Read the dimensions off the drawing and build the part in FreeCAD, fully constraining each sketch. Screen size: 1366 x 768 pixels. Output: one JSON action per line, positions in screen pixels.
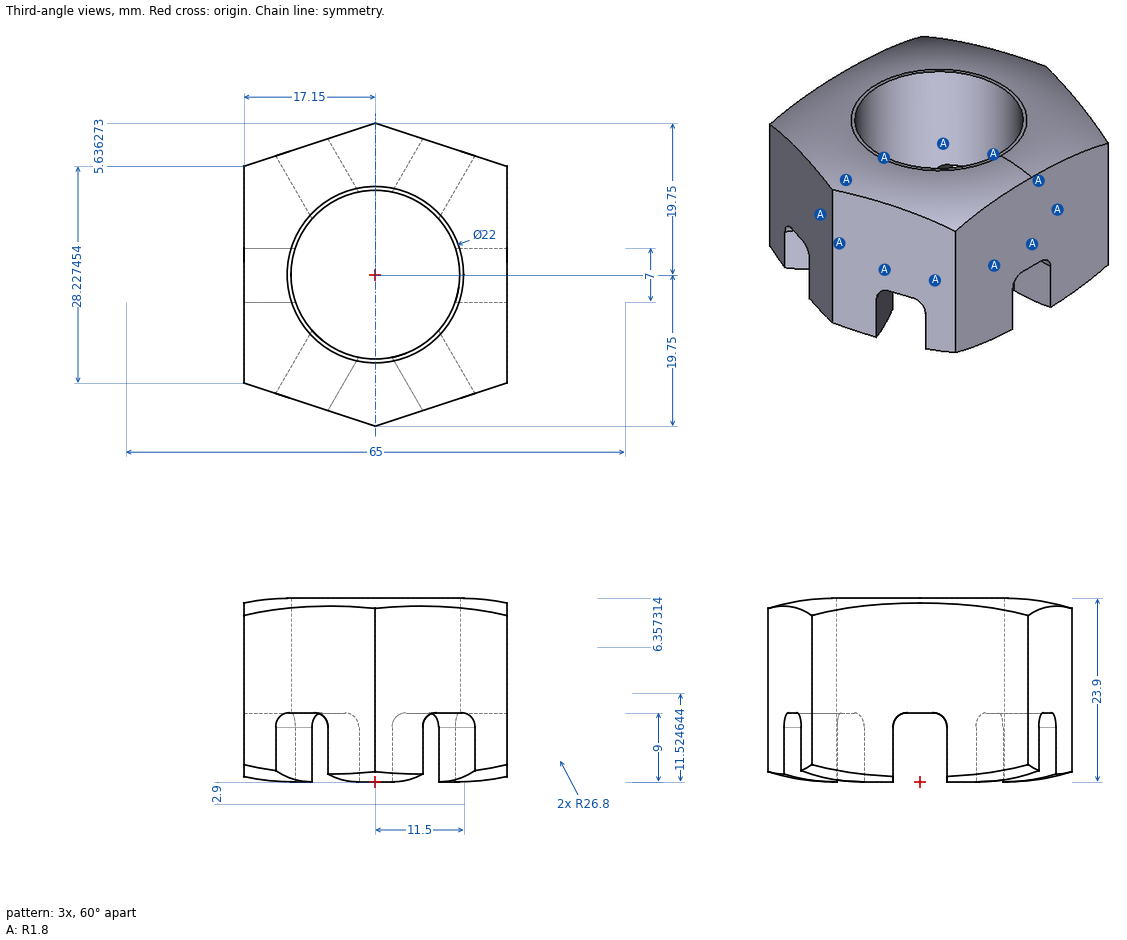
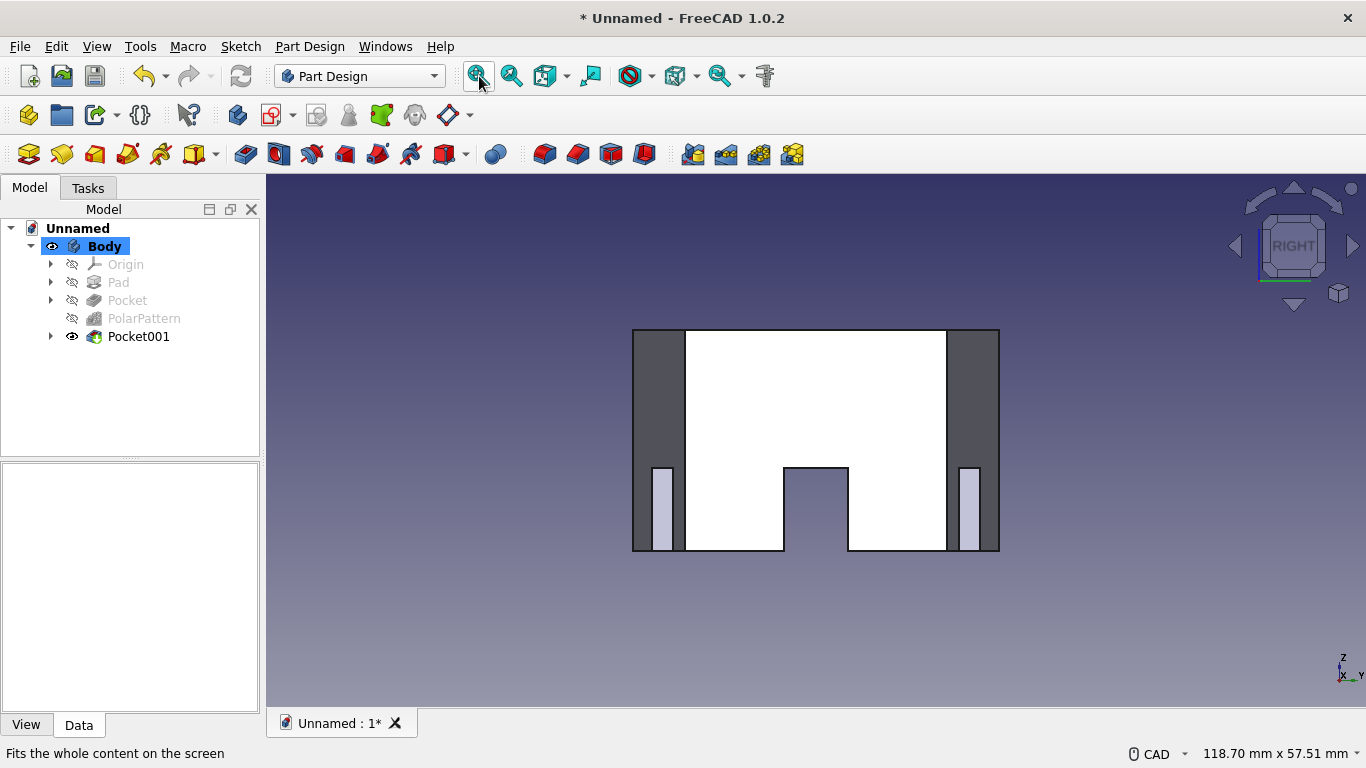
{"action": "key", "text": "5"}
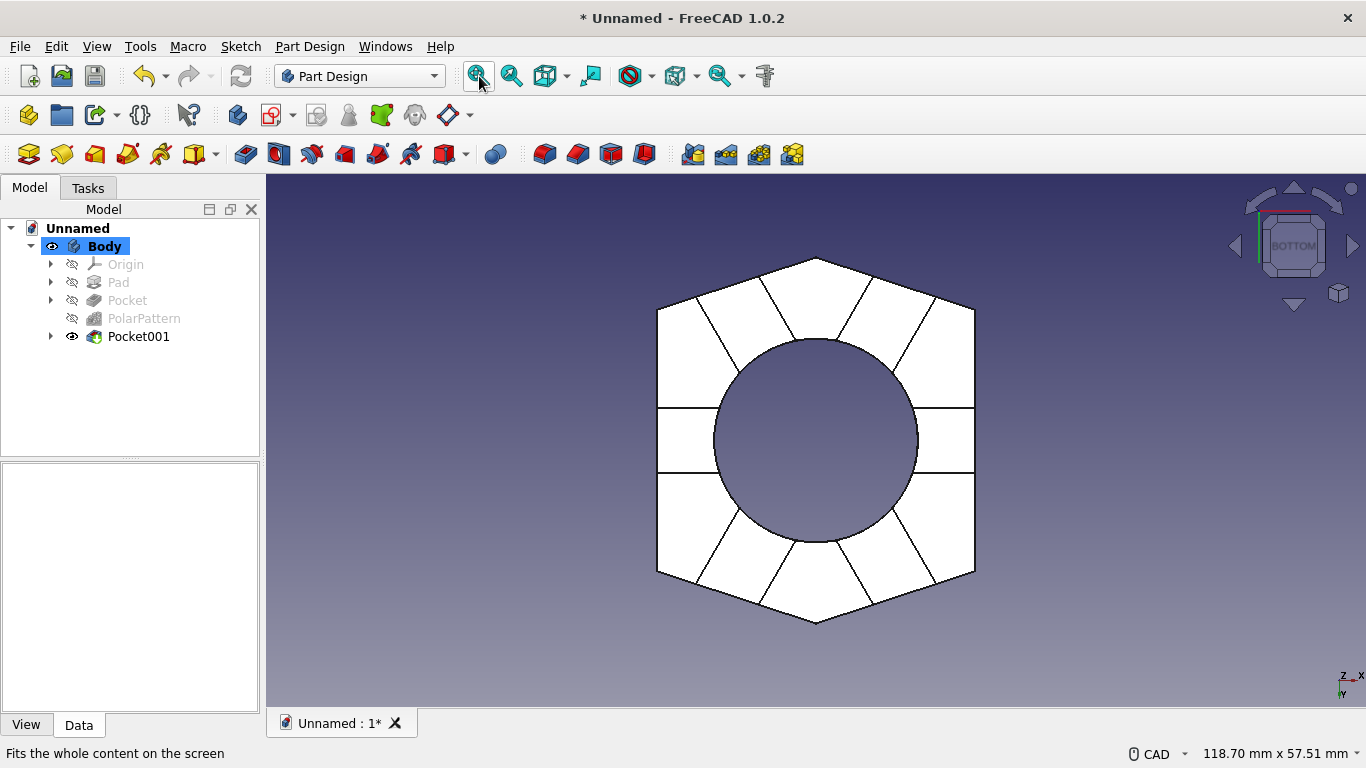
{"action": "key", "text": "4"}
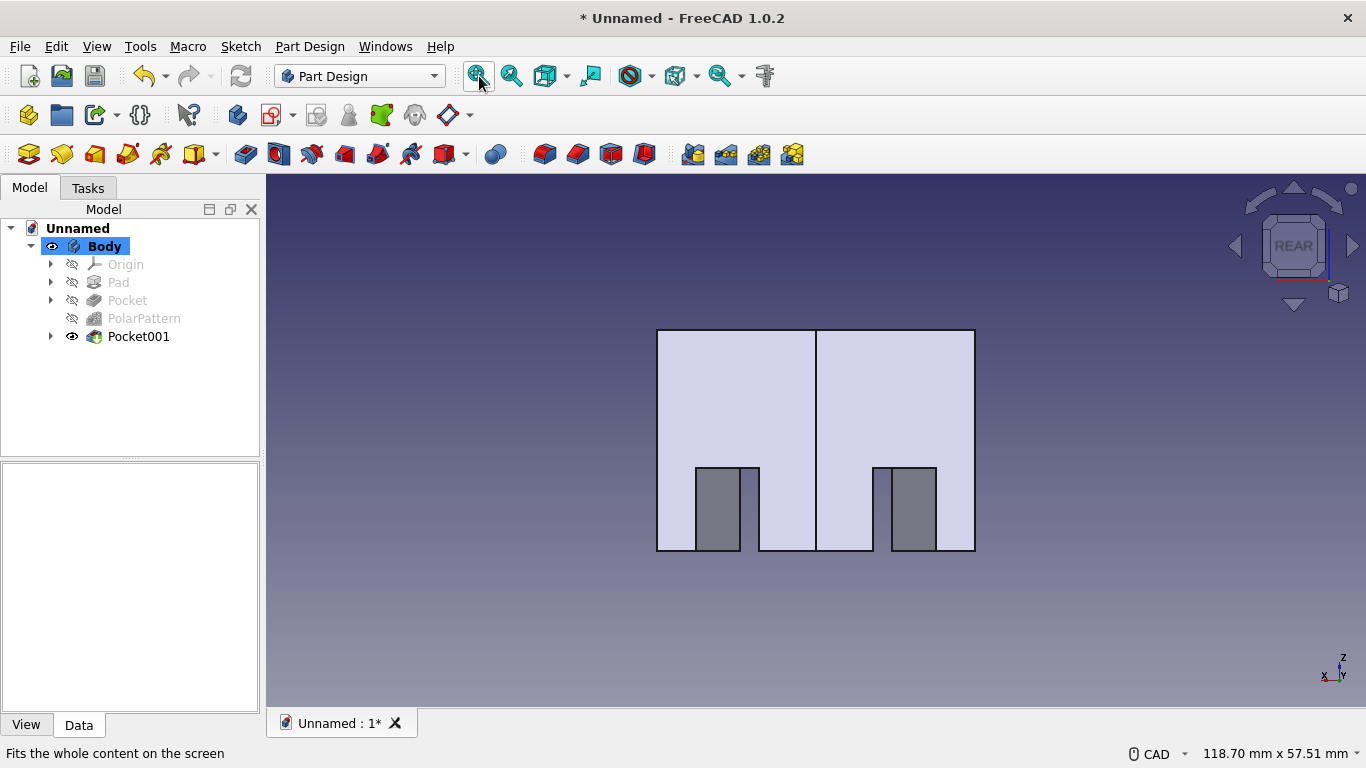
{"action": "left_click", "coordinate": [479, 76]}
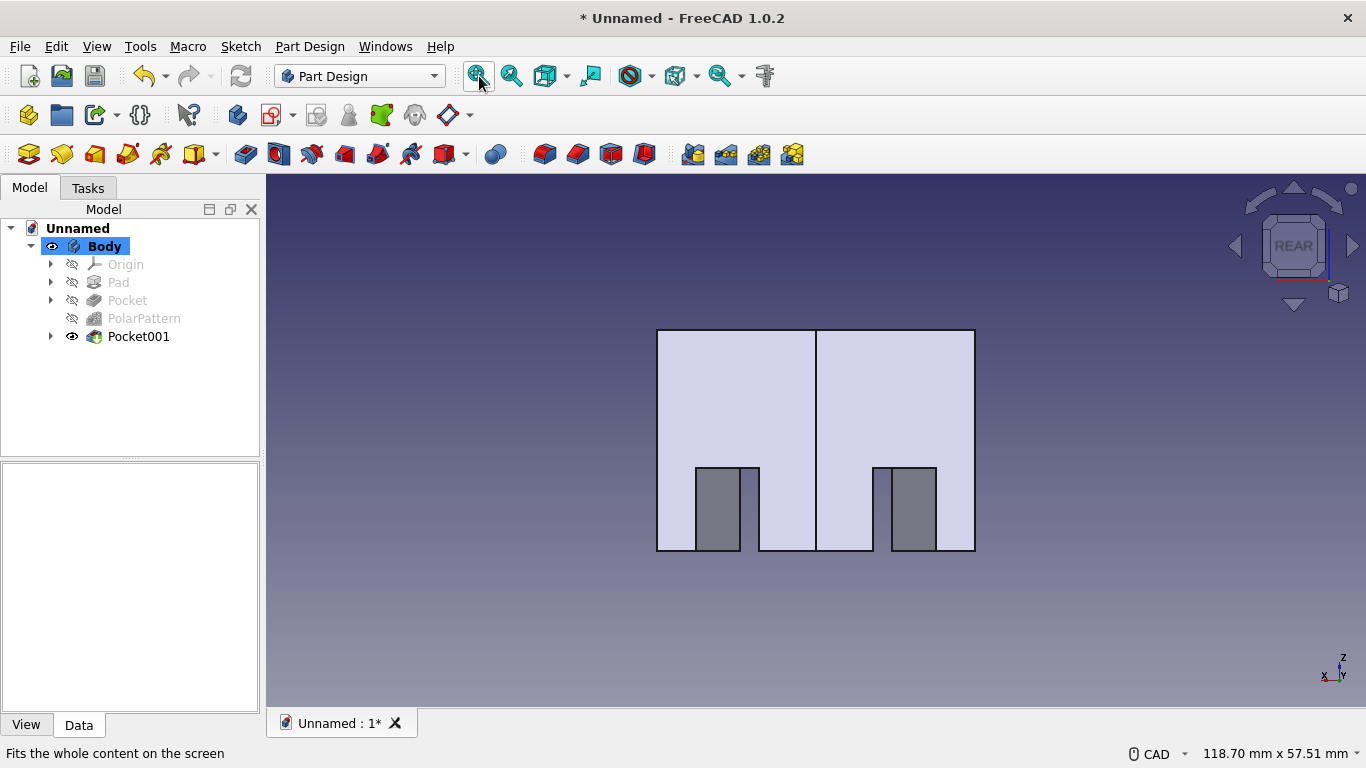
{"action": "key", "text": "6"}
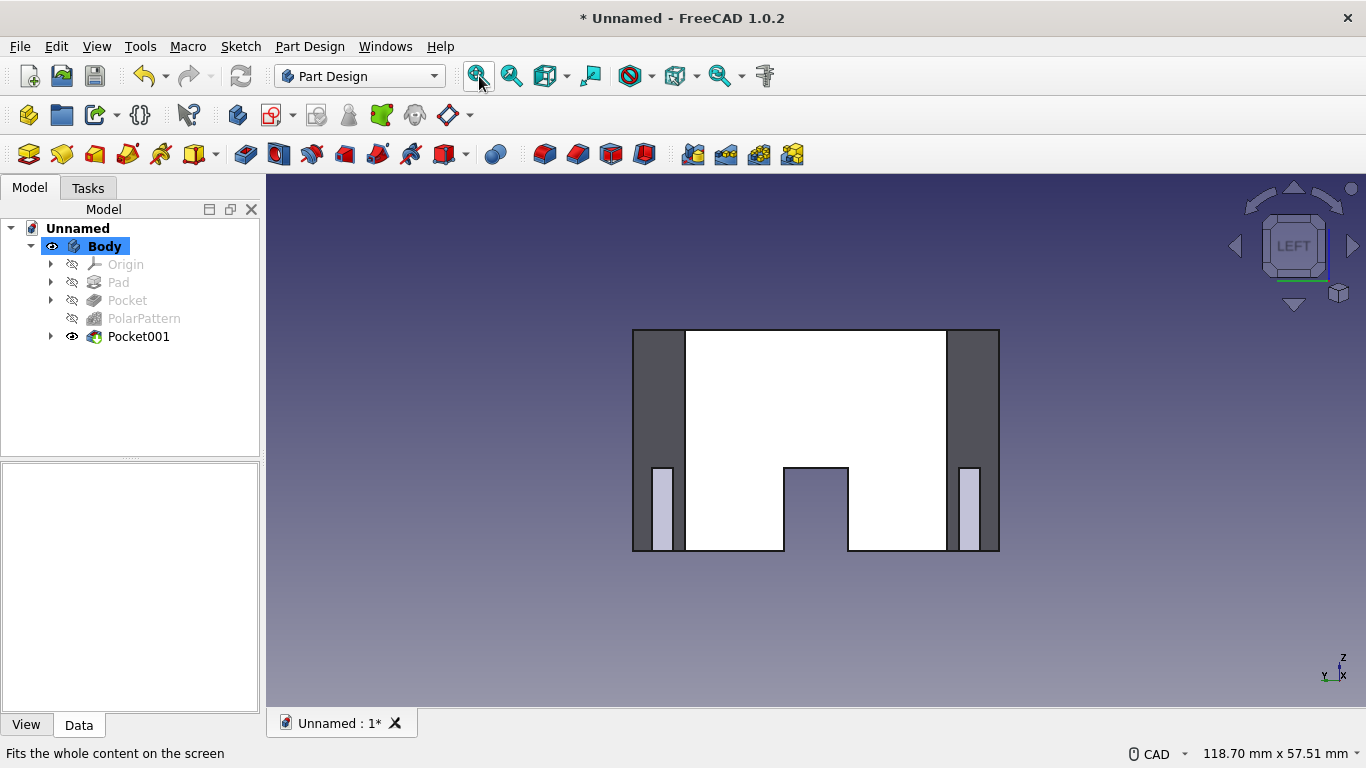
{"action": "left_click", "coordinate": [479, 76]}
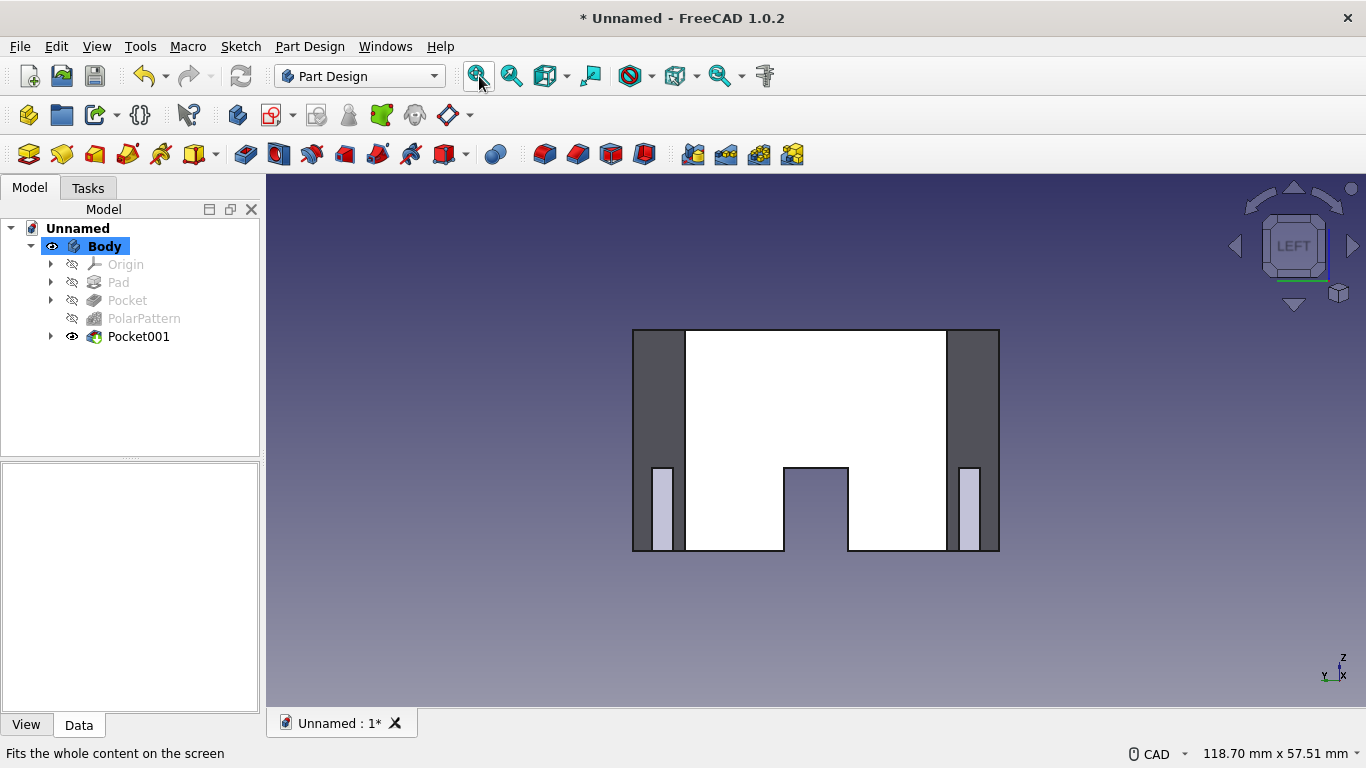
{"action": "key", "text": "v 3"}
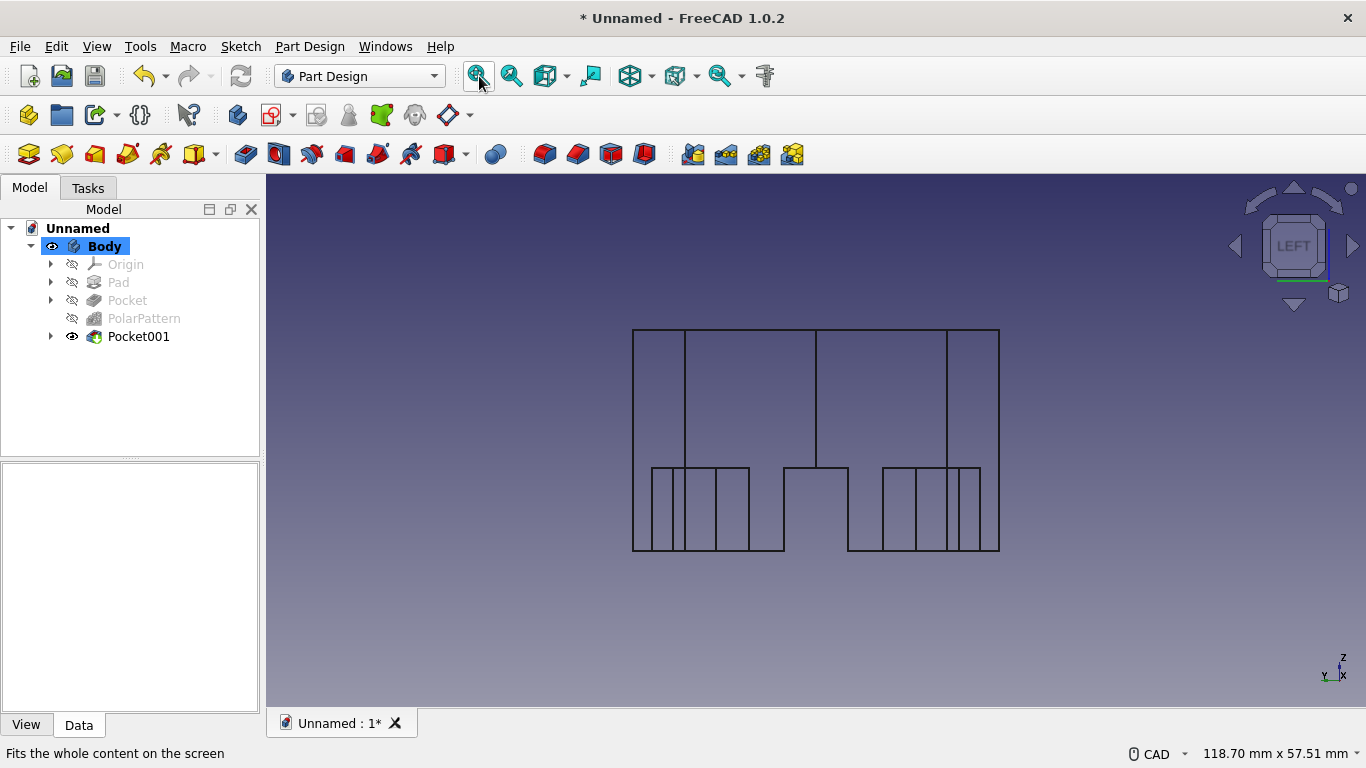
{"action": "key", "text": "0"}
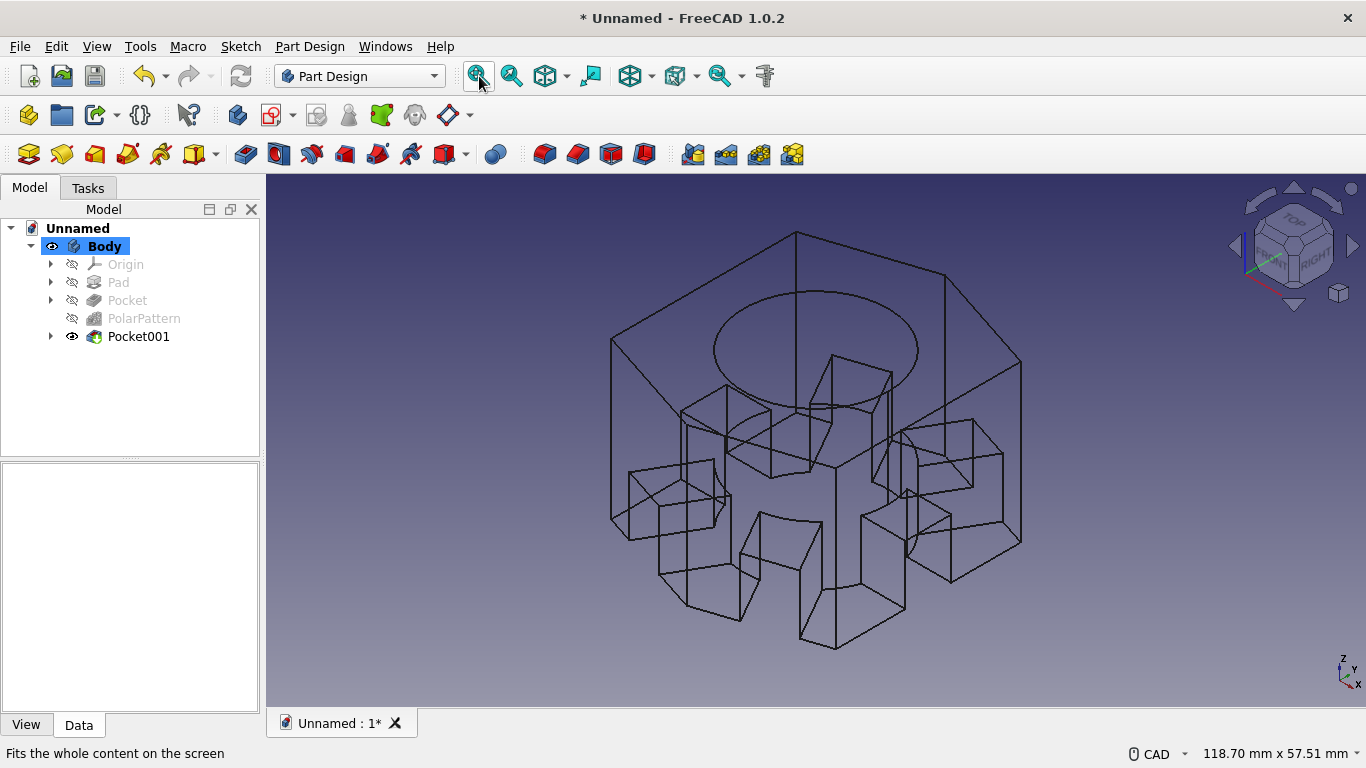
{"action": "left_click", "coordinate": [821, 379]}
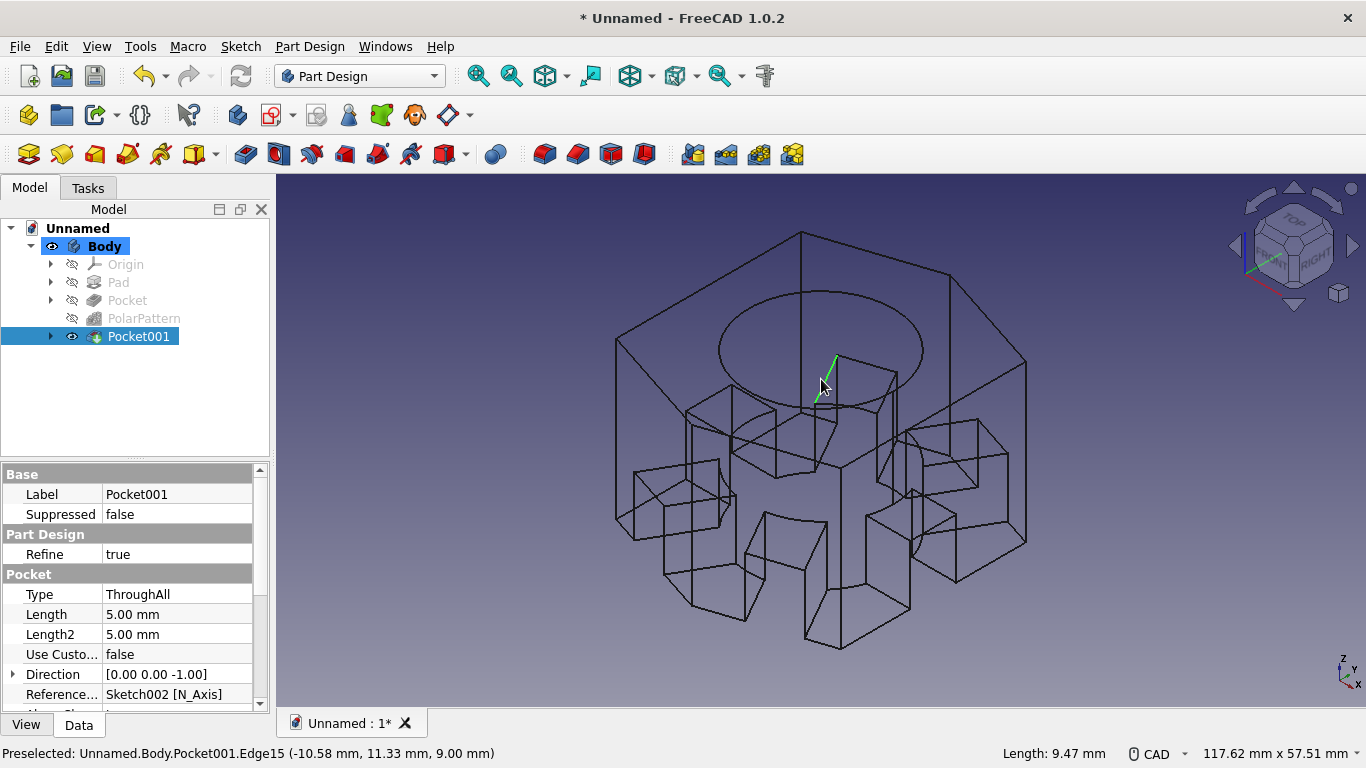
{"action": "left_click", "coordinate": [942, 424], "text": "ctrl"}